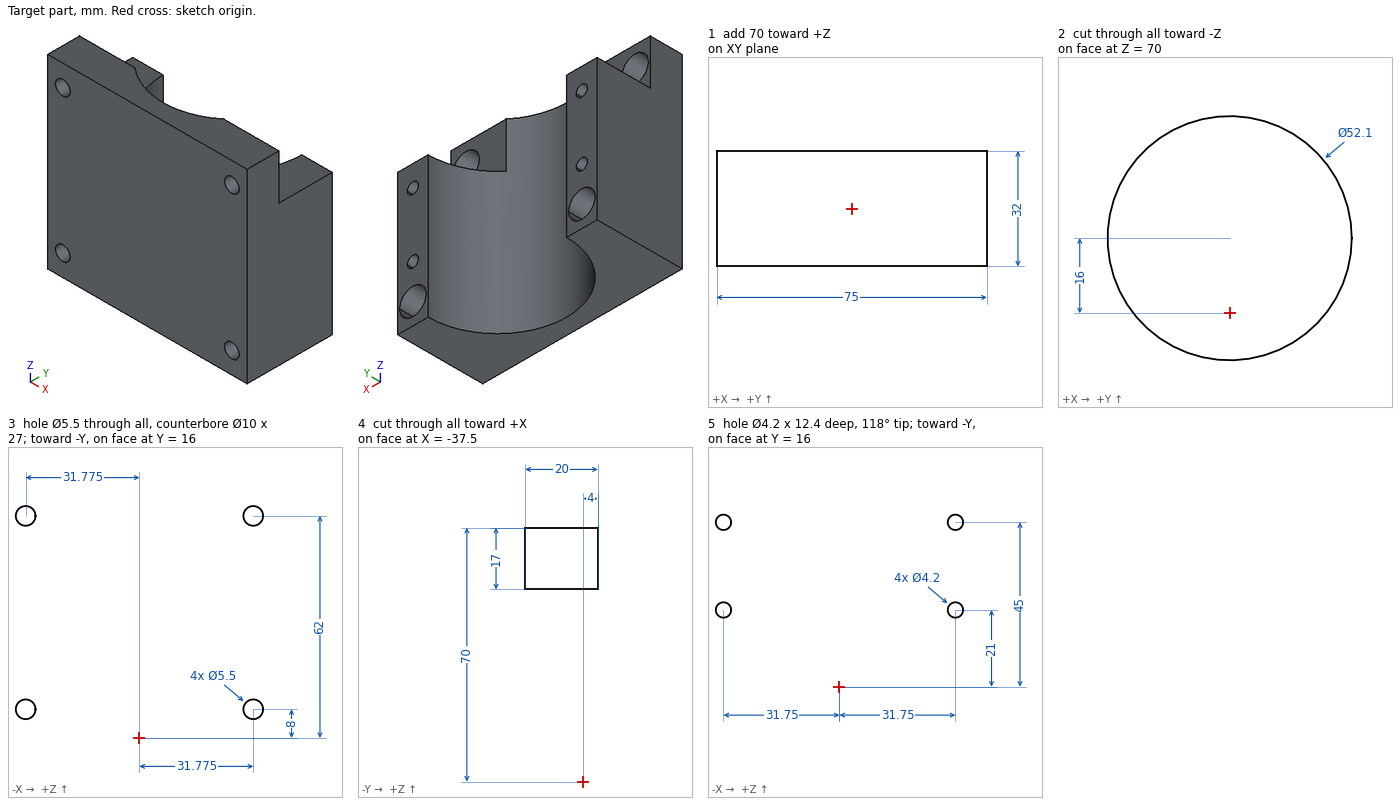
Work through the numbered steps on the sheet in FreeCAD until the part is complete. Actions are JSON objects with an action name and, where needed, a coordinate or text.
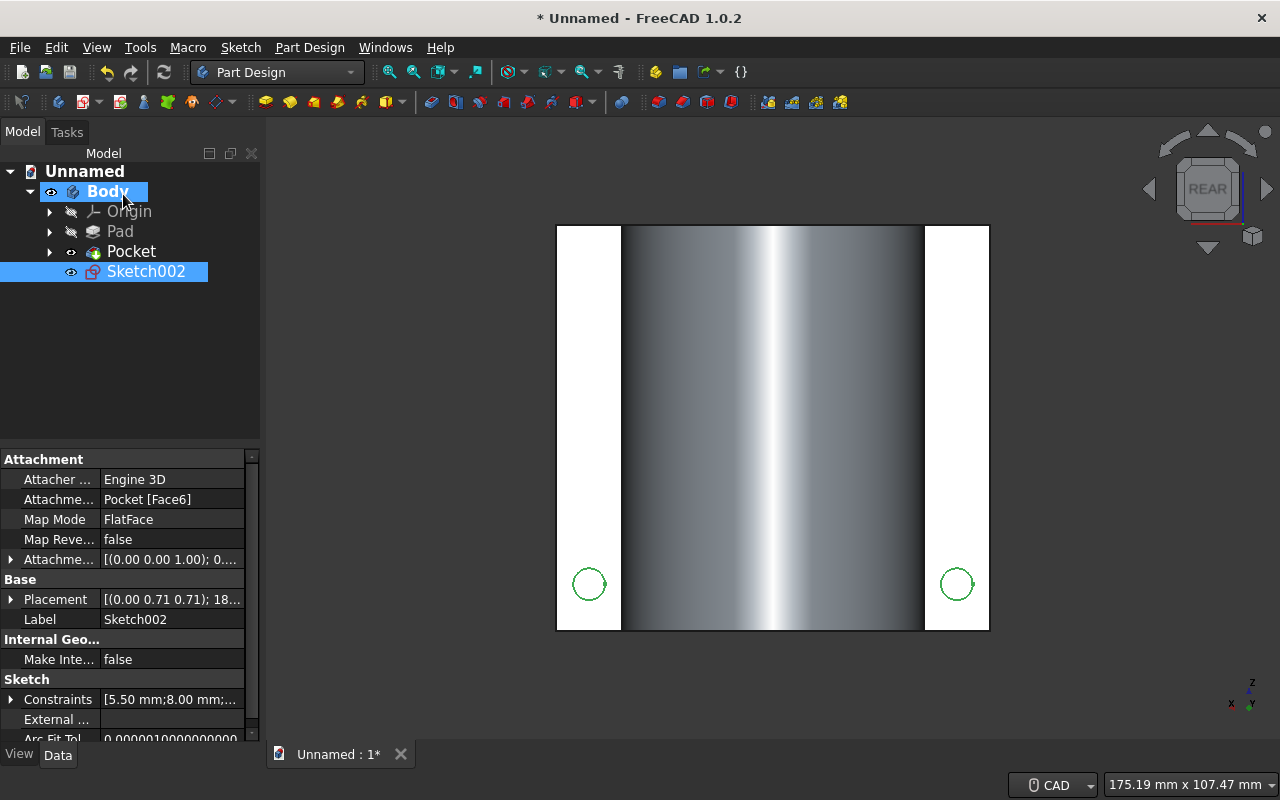
{"action": "left_click", "coordinate": [456, 102]}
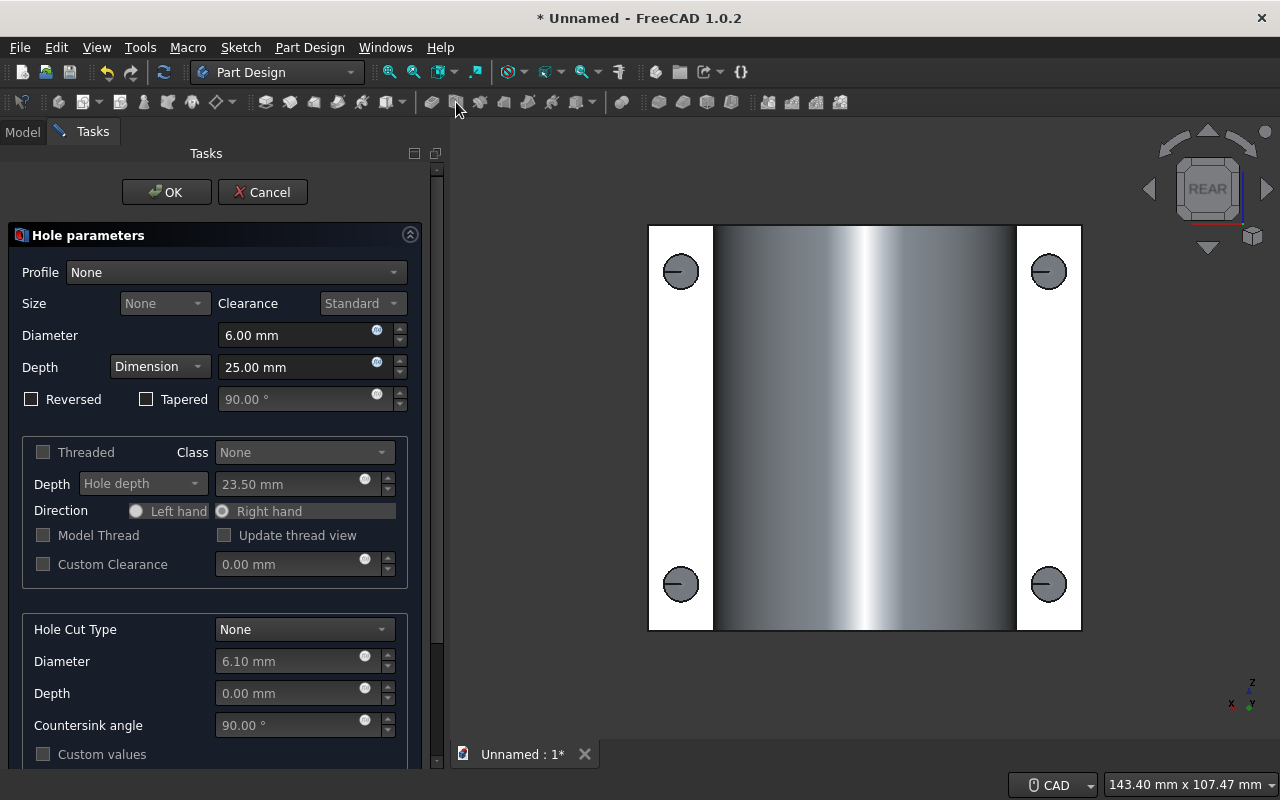
{"action": "triple_click", "coordinate": [305, 335]}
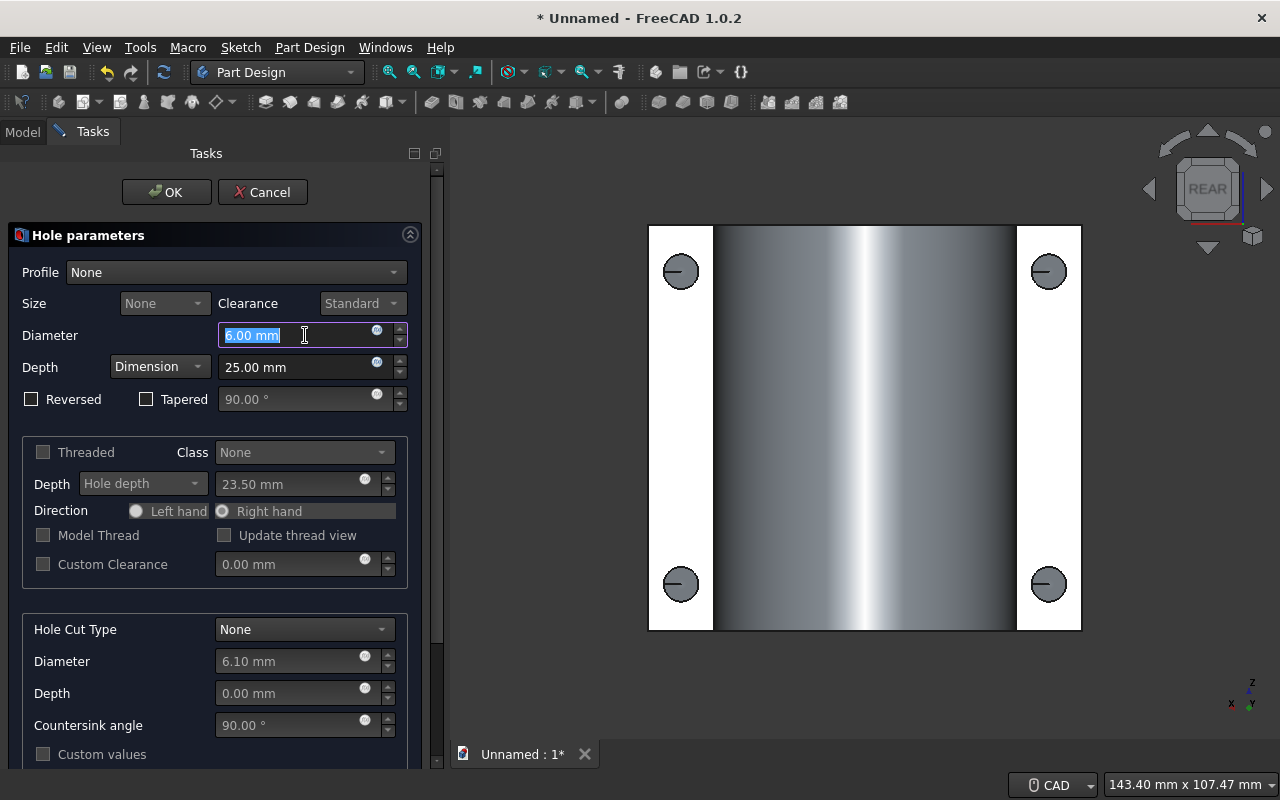
{"action": "type", "text": "5.5"}
{"action": "key", "text": "Tab"}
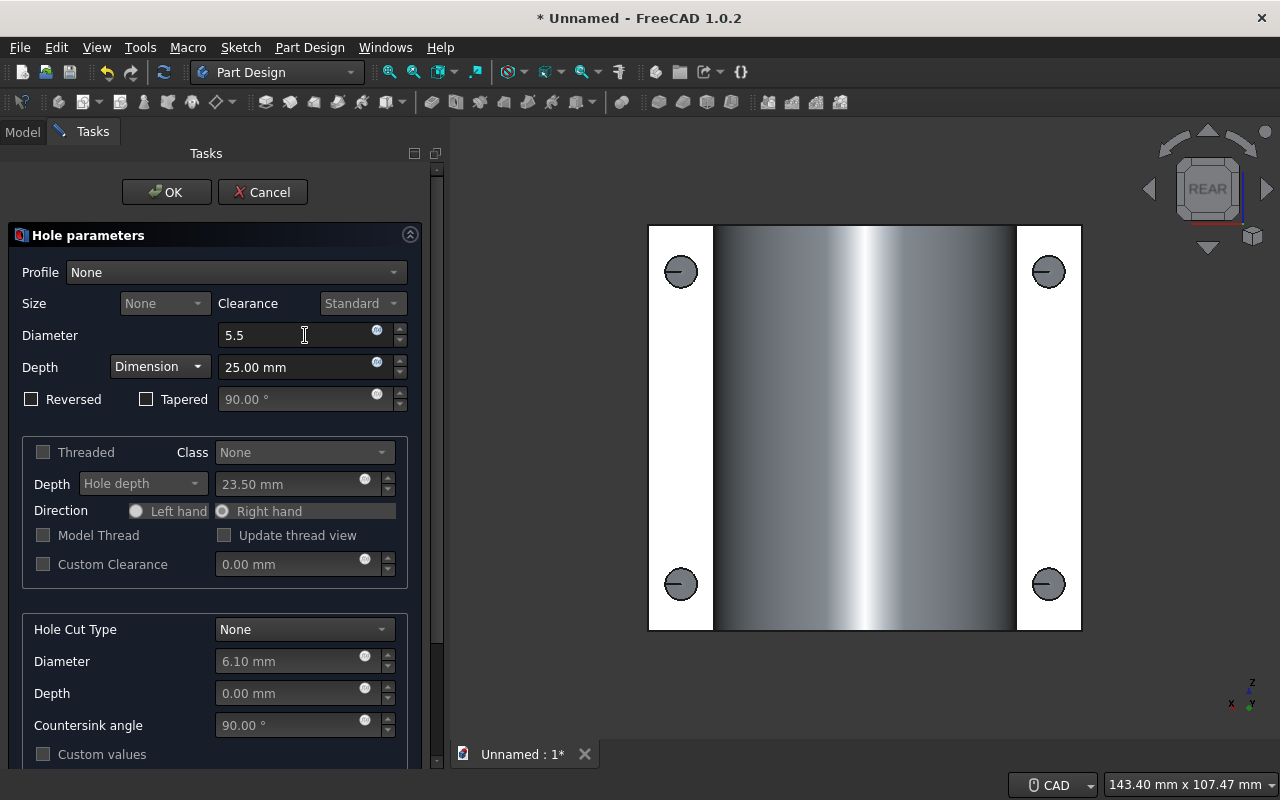
{"action": "left_click", "coordinate": [161, 366]}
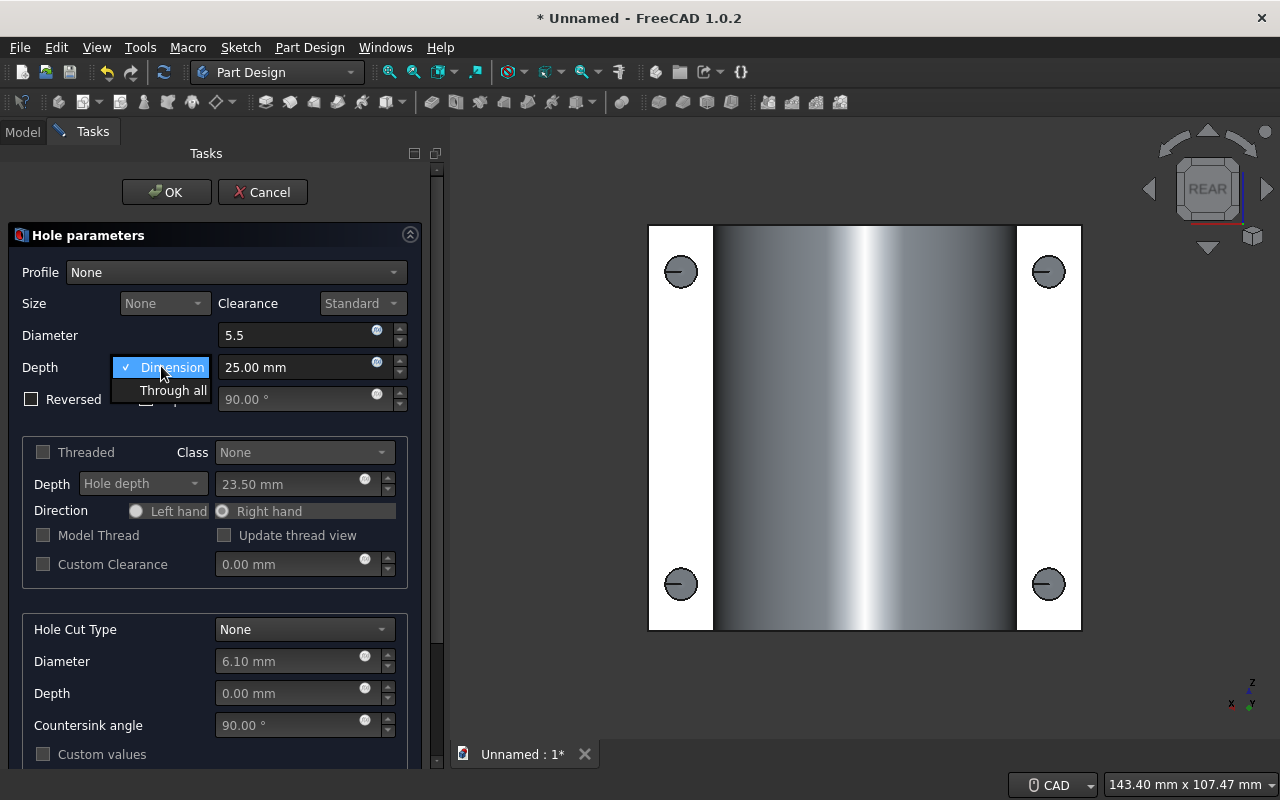
{"action": "left_click", "coordinate": [160, 390]}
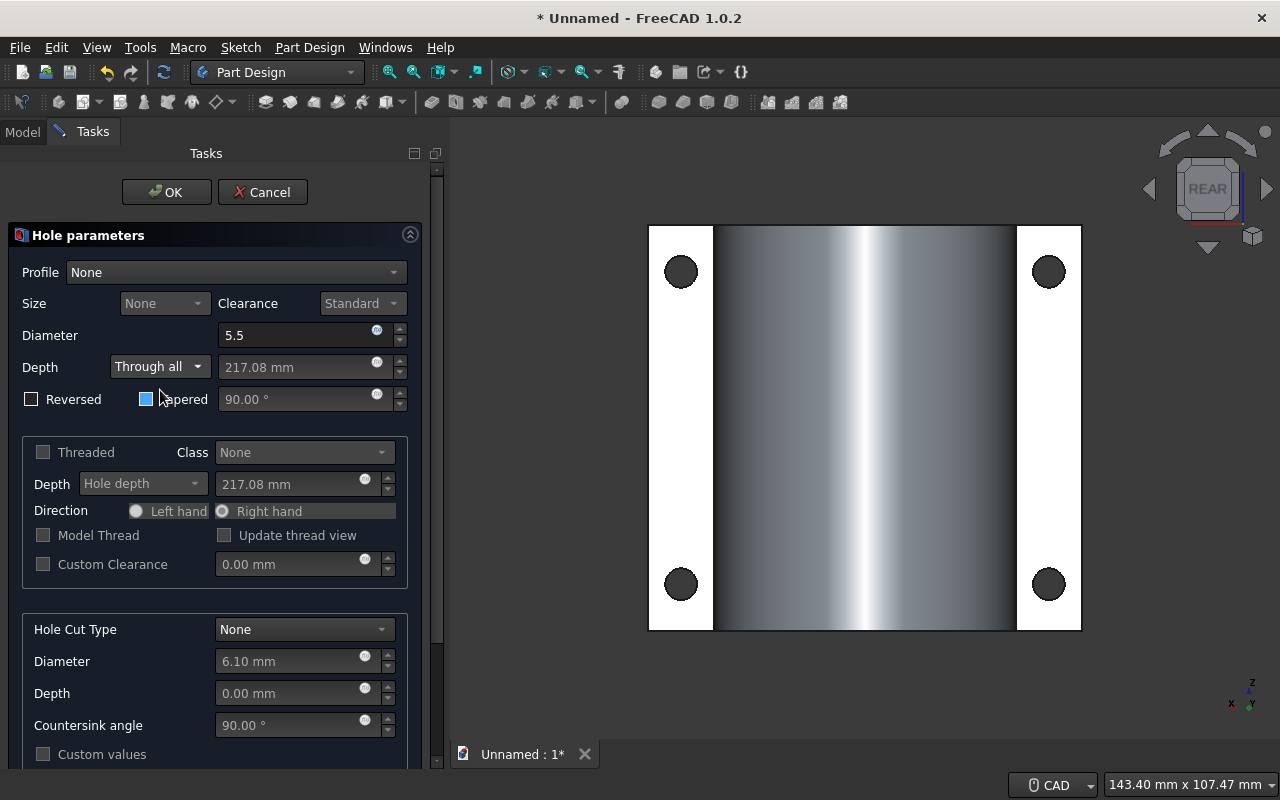
{"action": "left_click", "coordinate": [306, 630]}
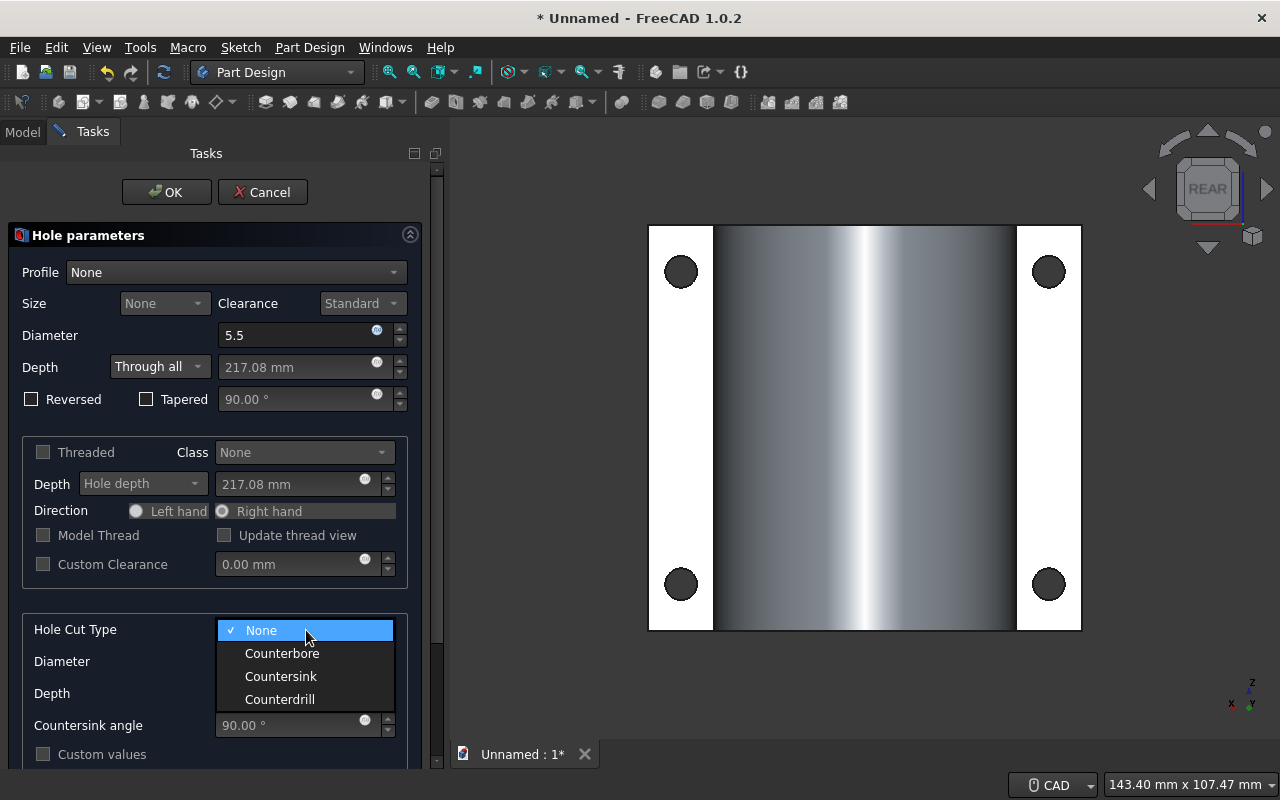
{"action": "left_click", "coordinate": [304, 654]}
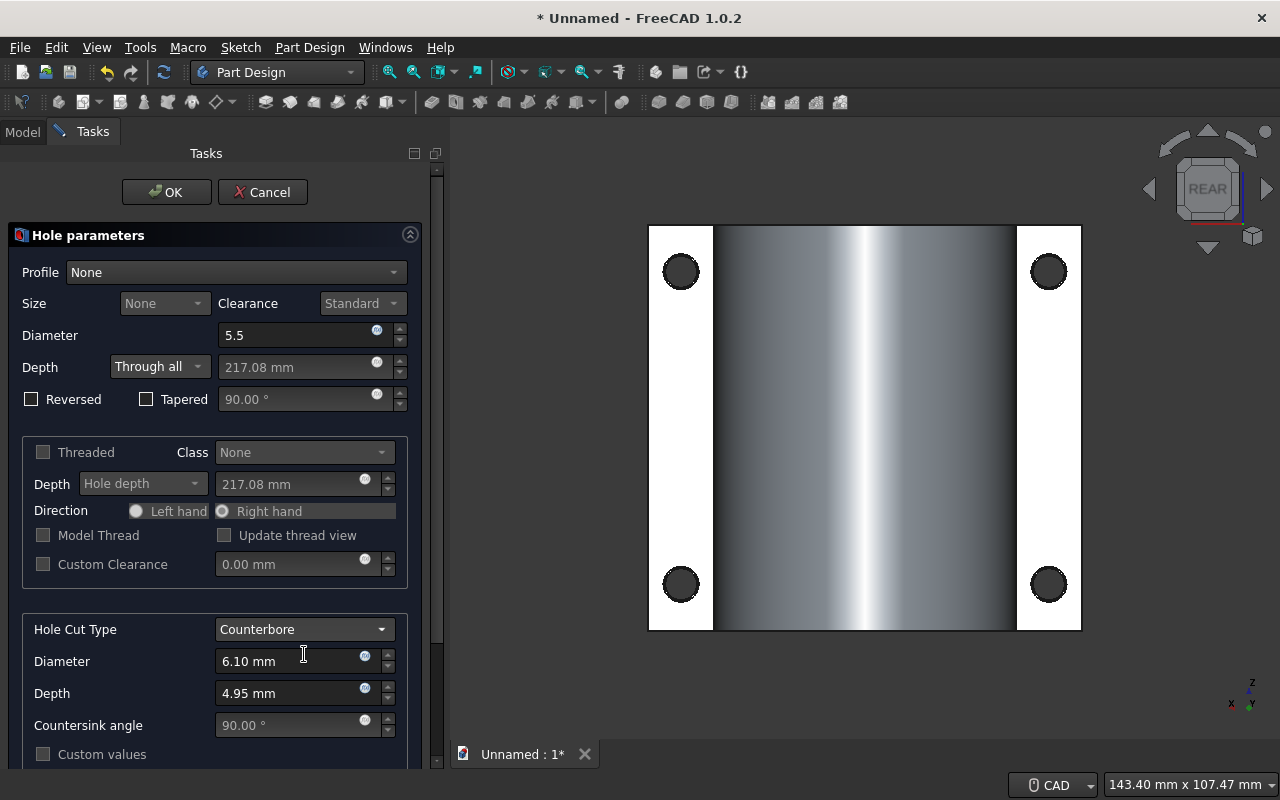
{"action": "triple_click", "coordinate": [298, 661]}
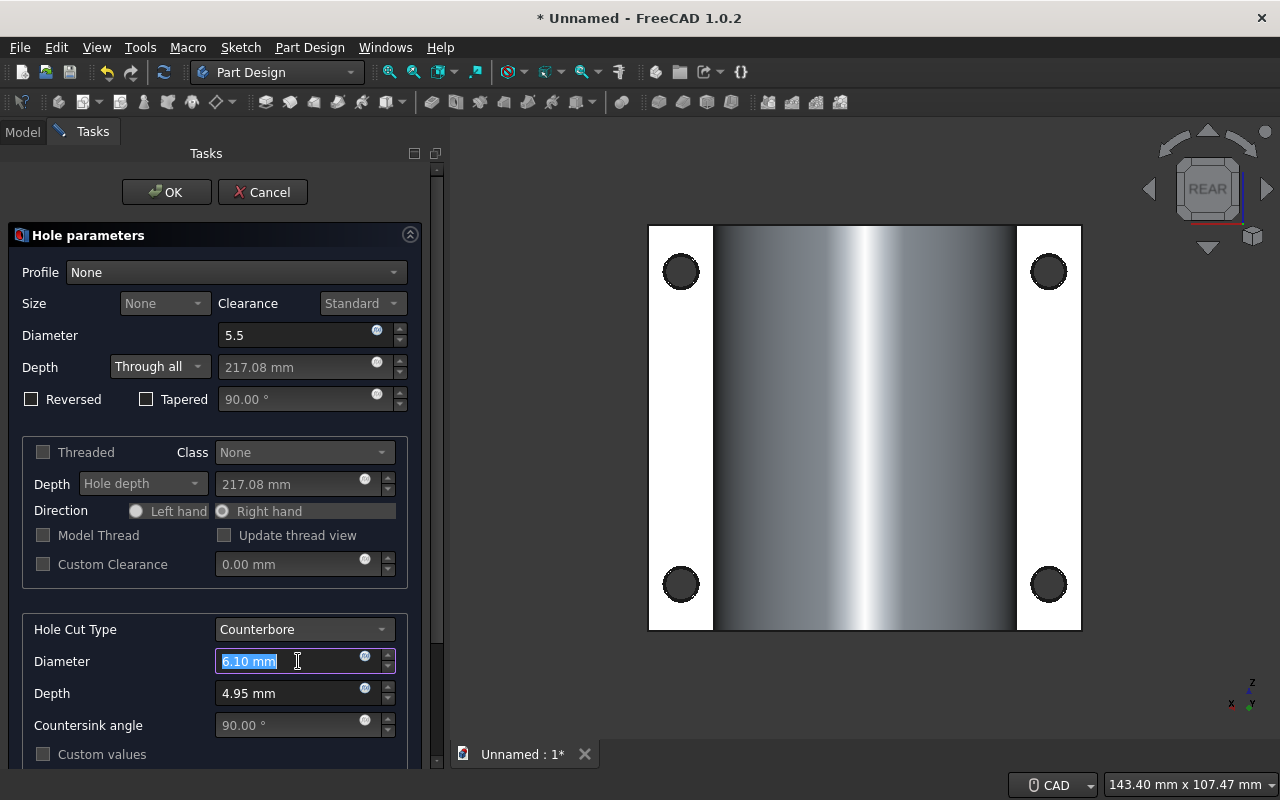
{"action": "type", "text": "10"}
{"action": "key", "text": "Tab"}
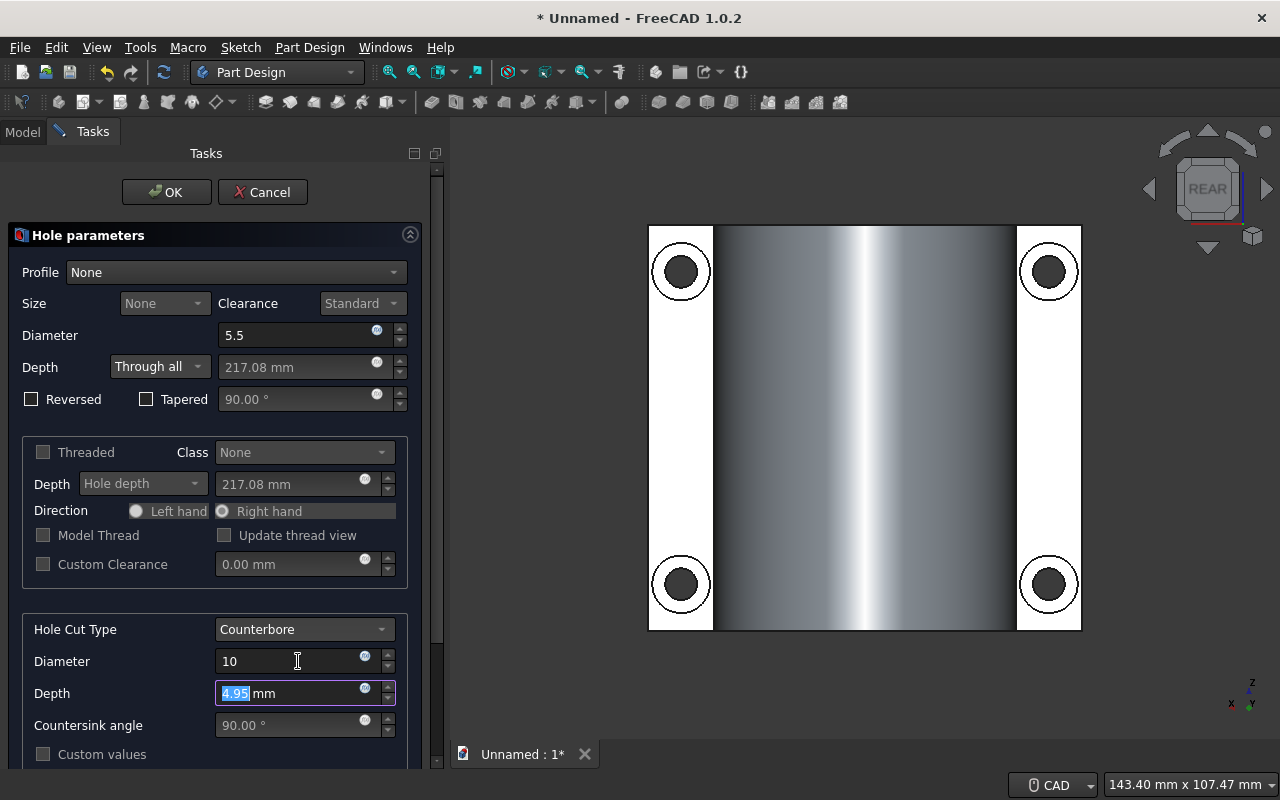
{"action": "type", "text": "27"}
{"action": "key", "text": "Tab"}